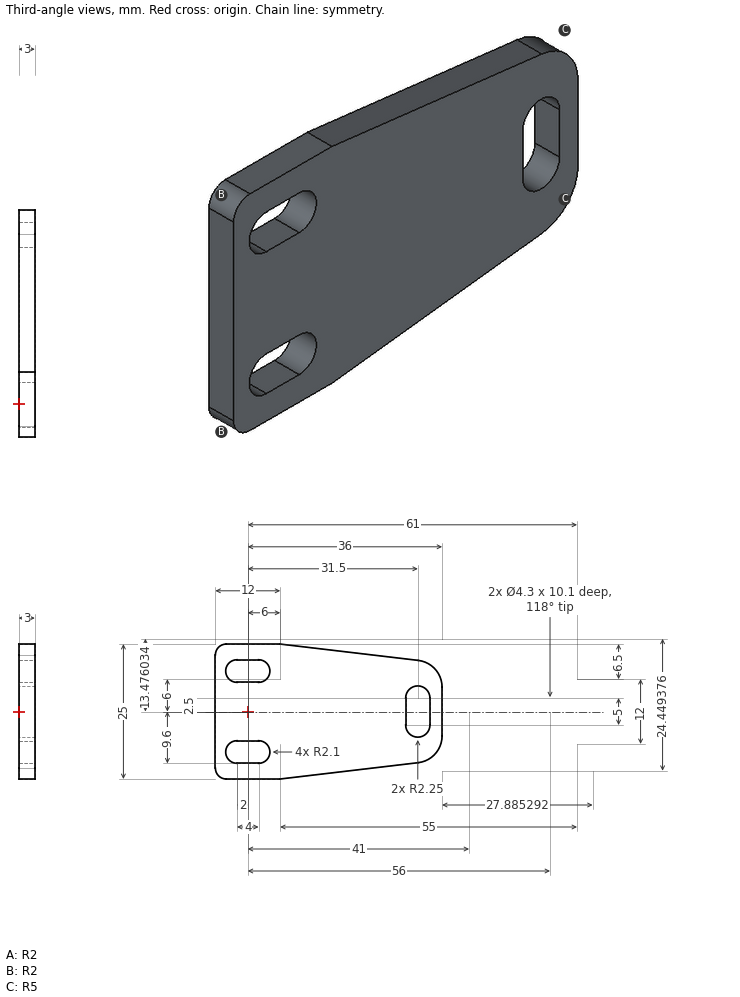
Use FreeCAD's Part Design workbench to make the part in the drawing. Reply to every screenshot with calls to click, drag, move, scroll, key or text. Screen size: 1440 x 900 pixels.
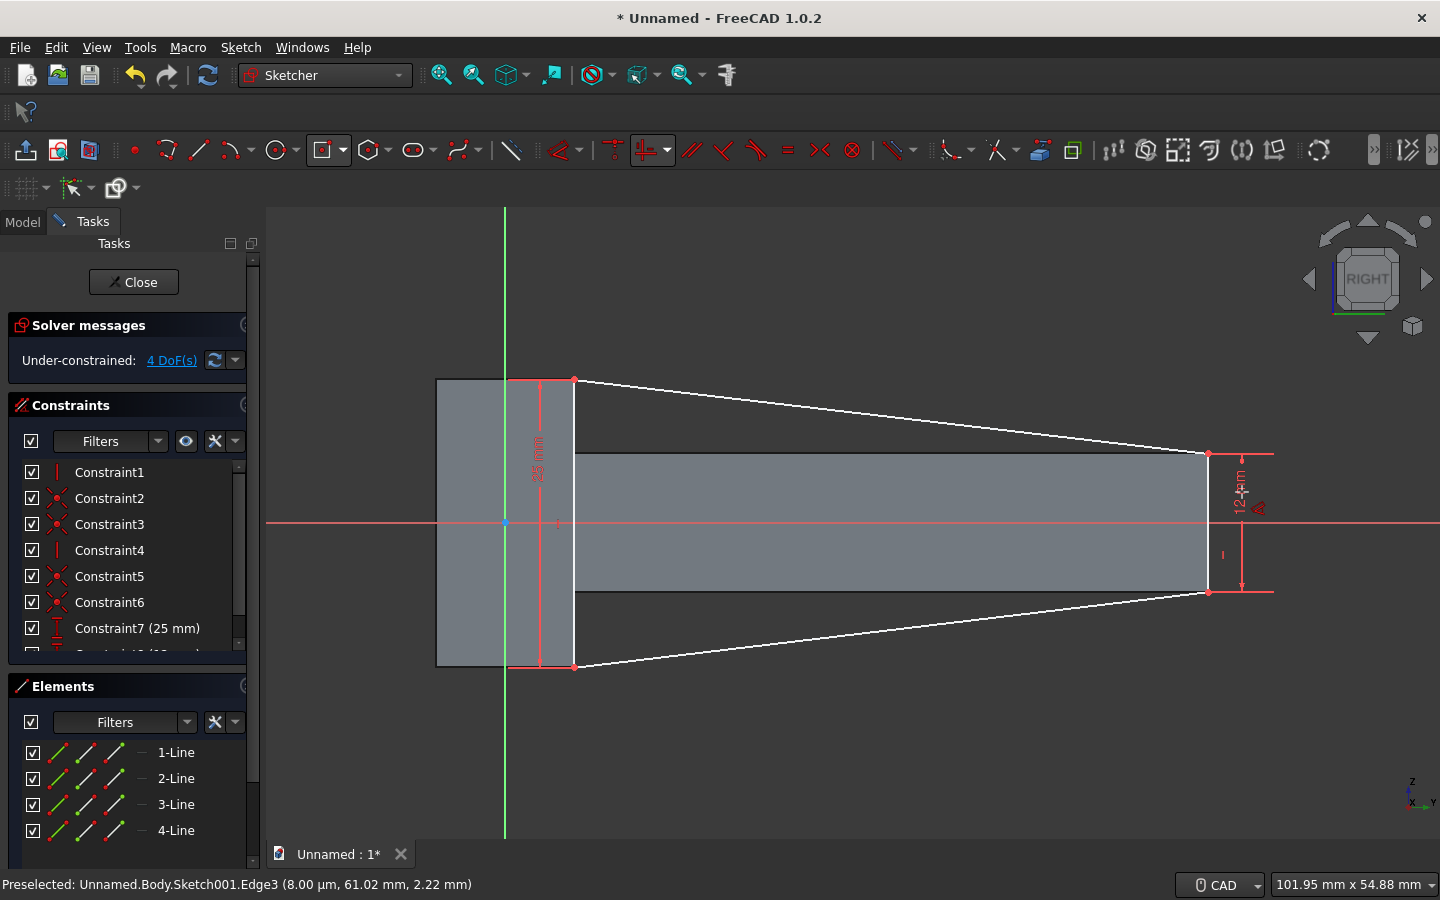
click(574, 668)
click(540, 702)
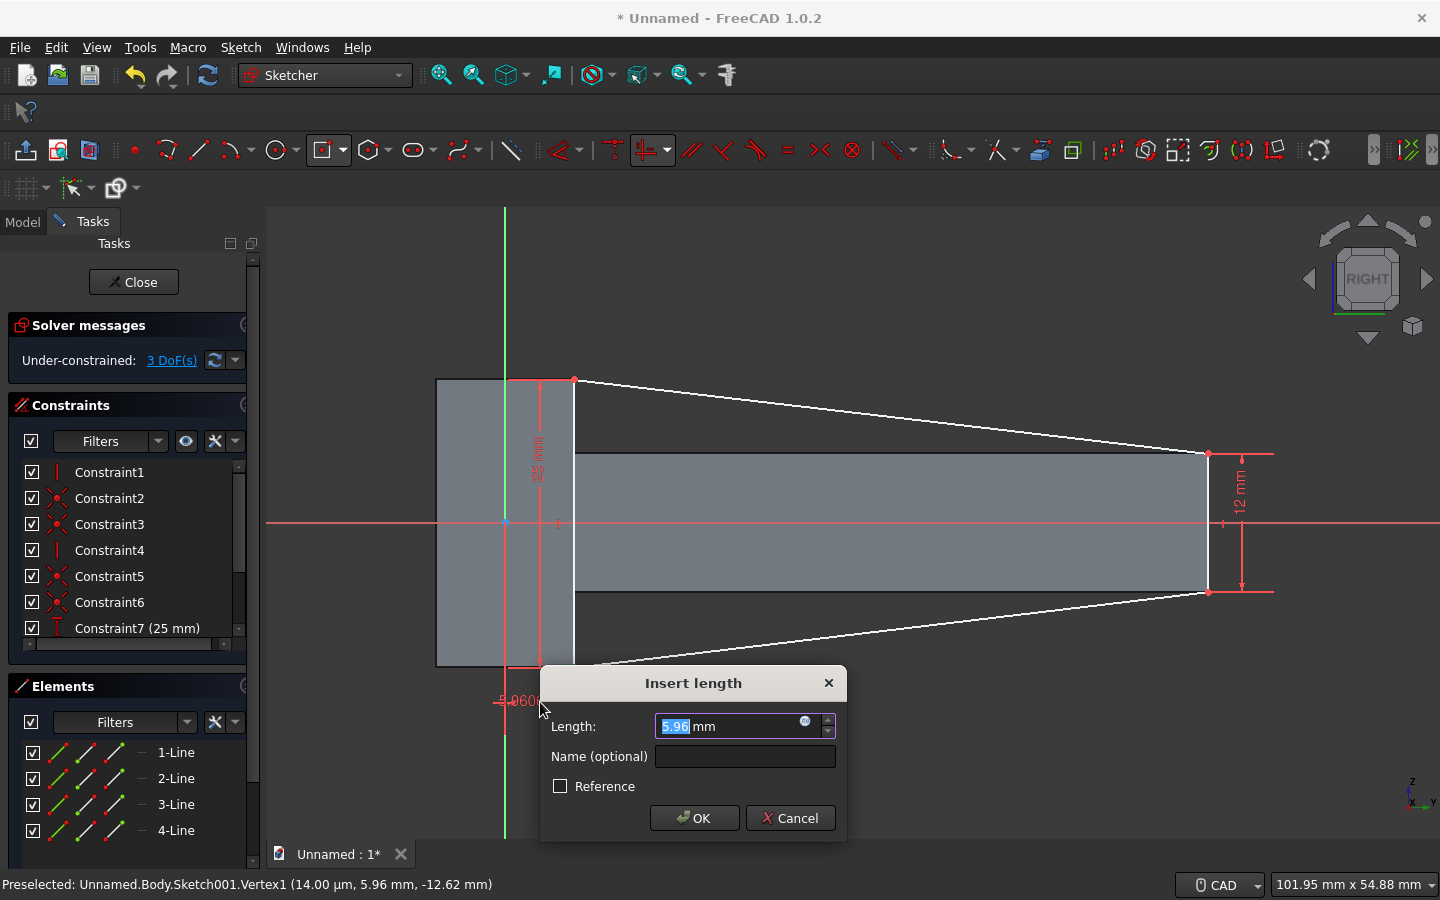
text(6)
key(Return)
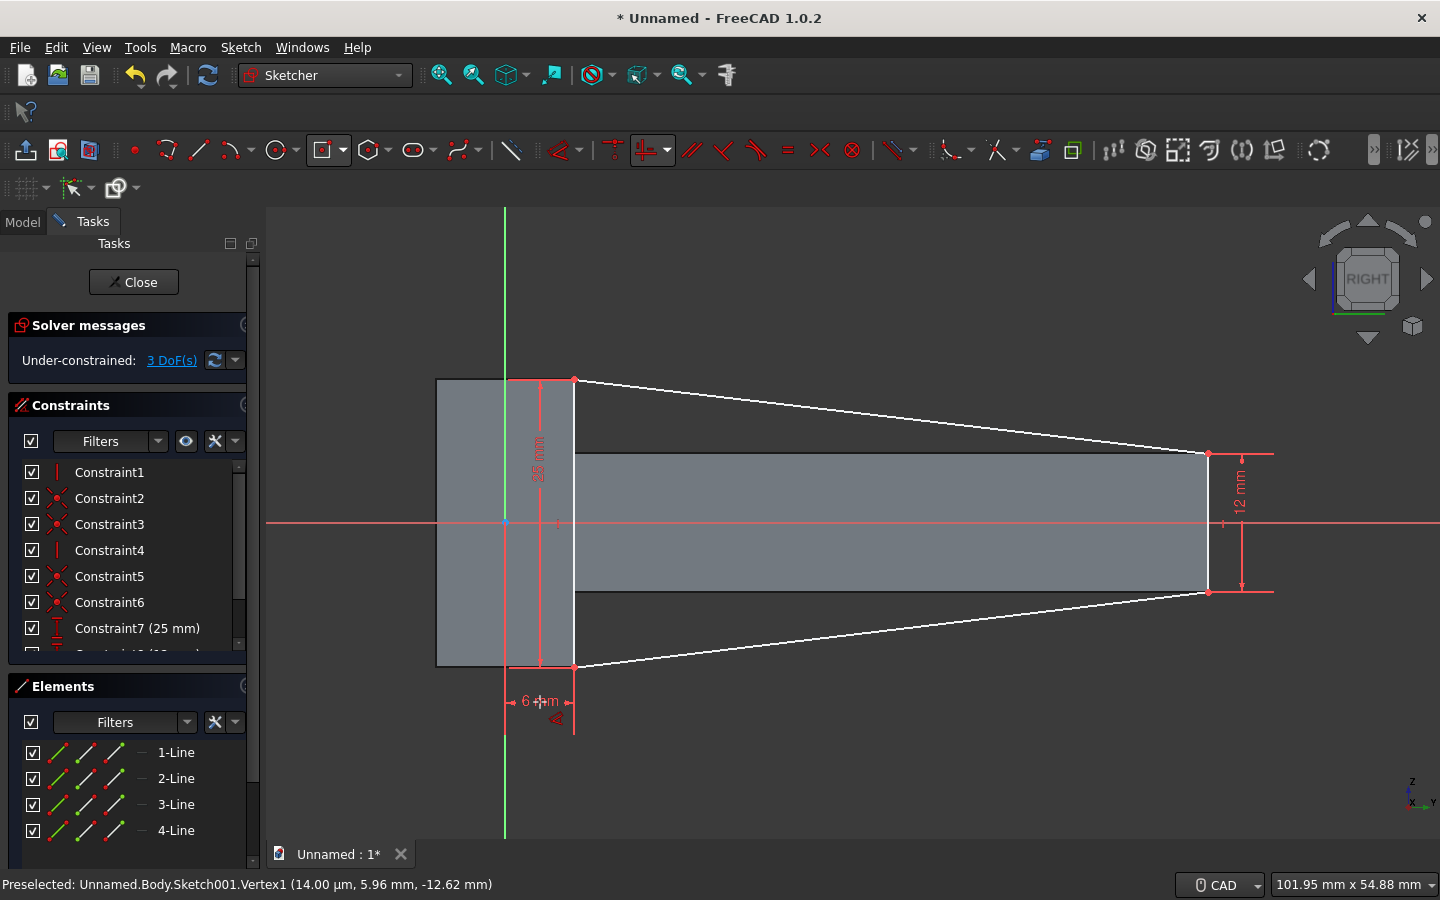
click(1208, 454)
click(1242, 464)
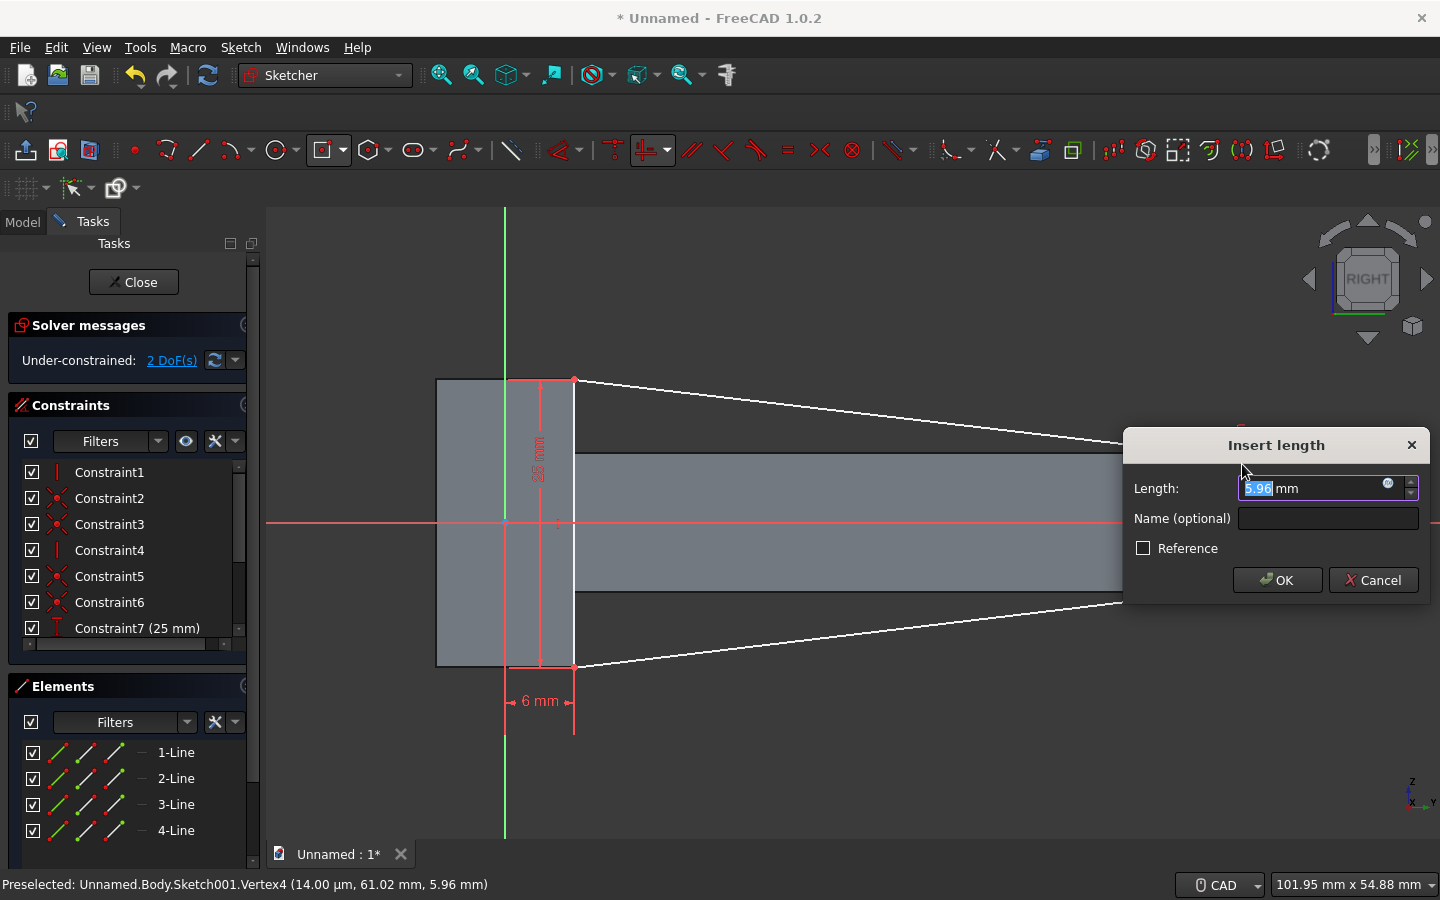
text(6)
key(Return)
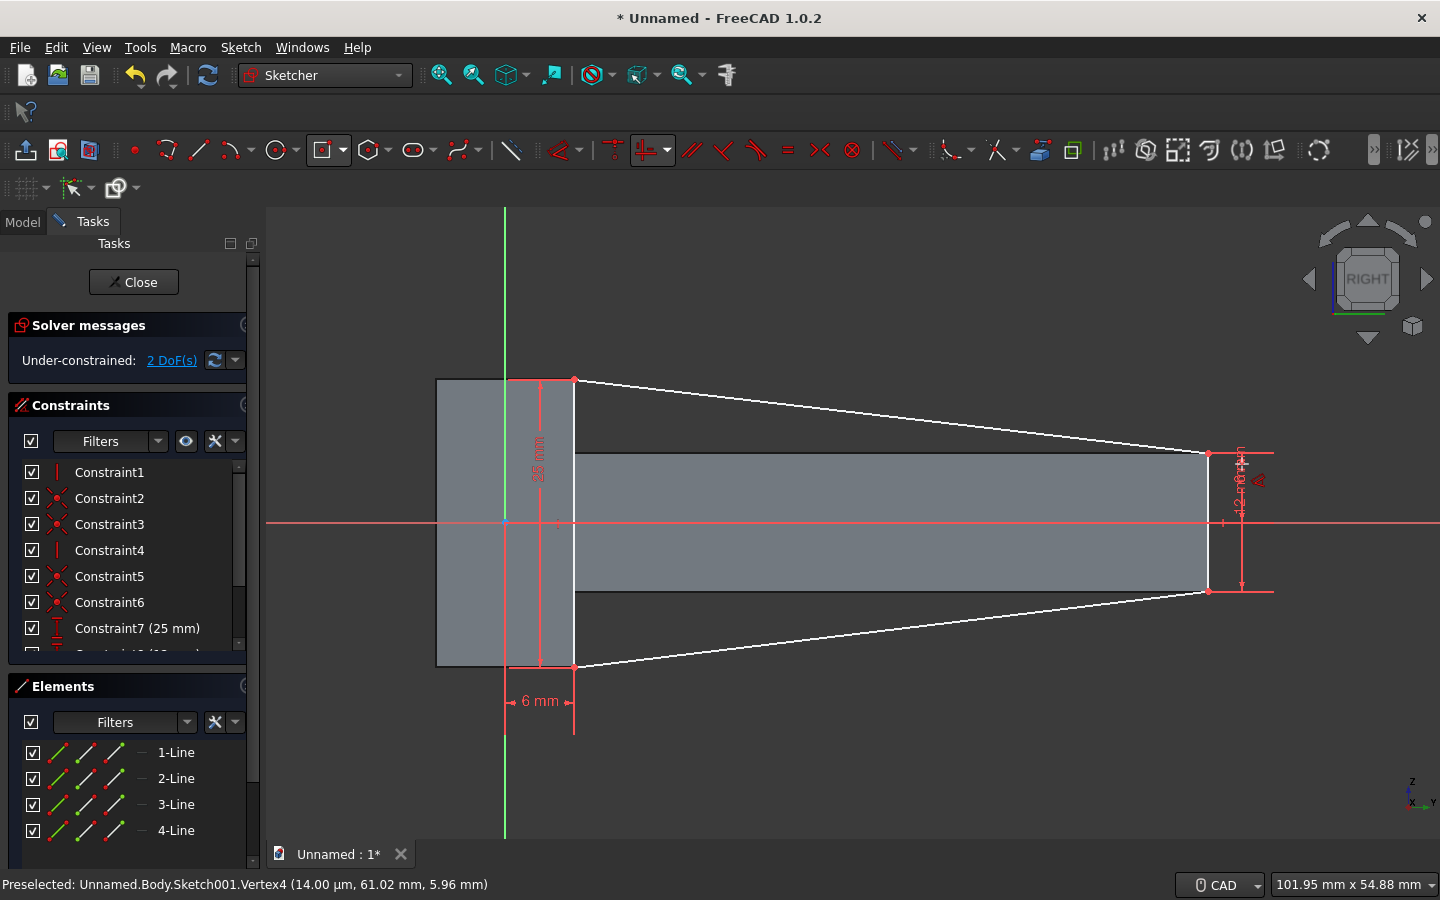
click(1208, 453)
click(695, 419)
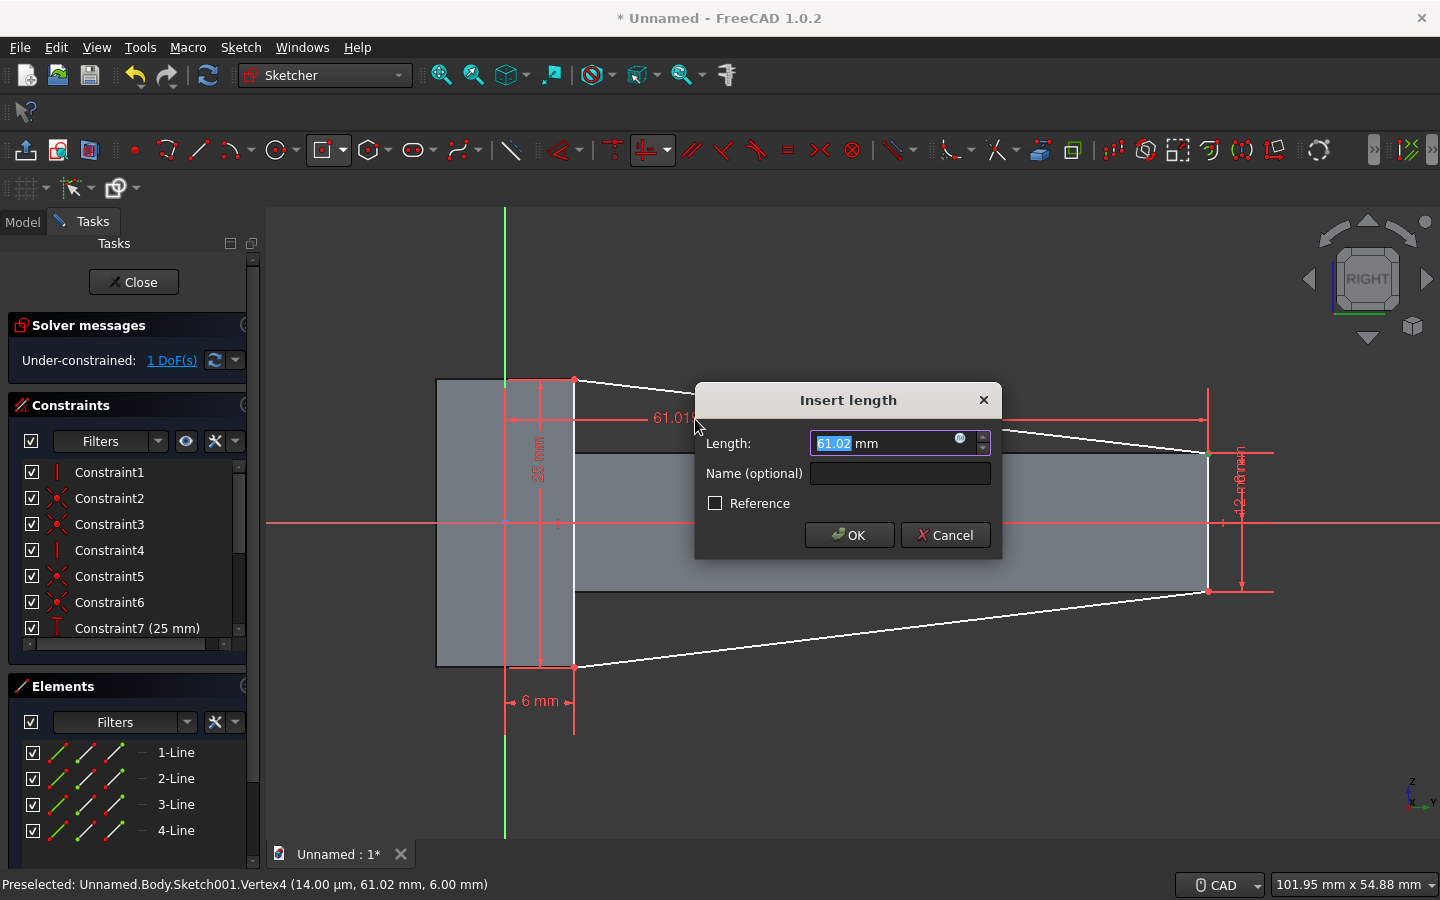
text(61)
key(Return)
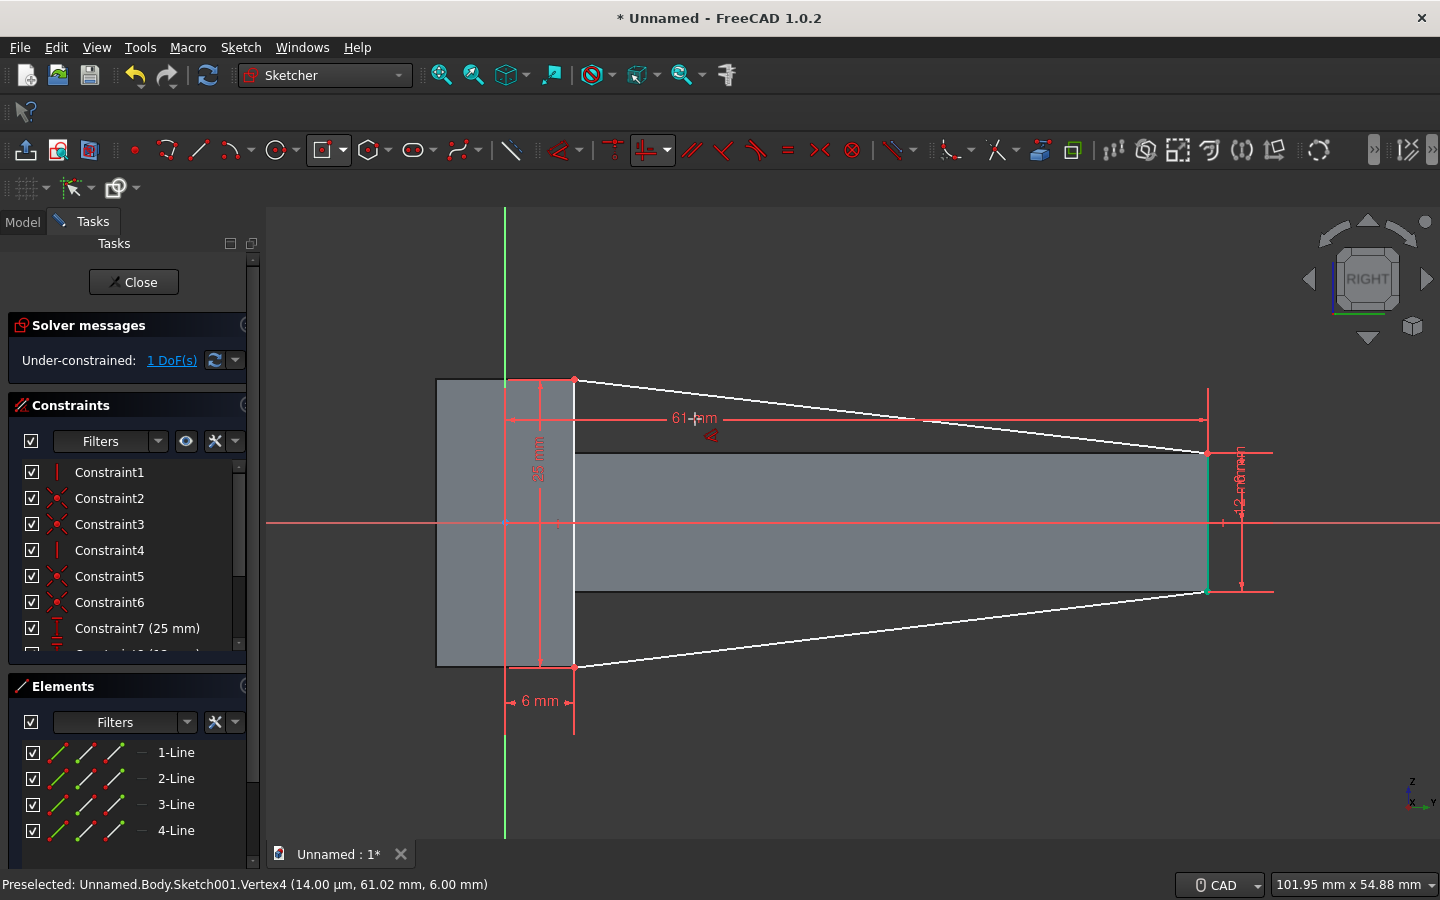
click(764, 402)
click(1242, 417)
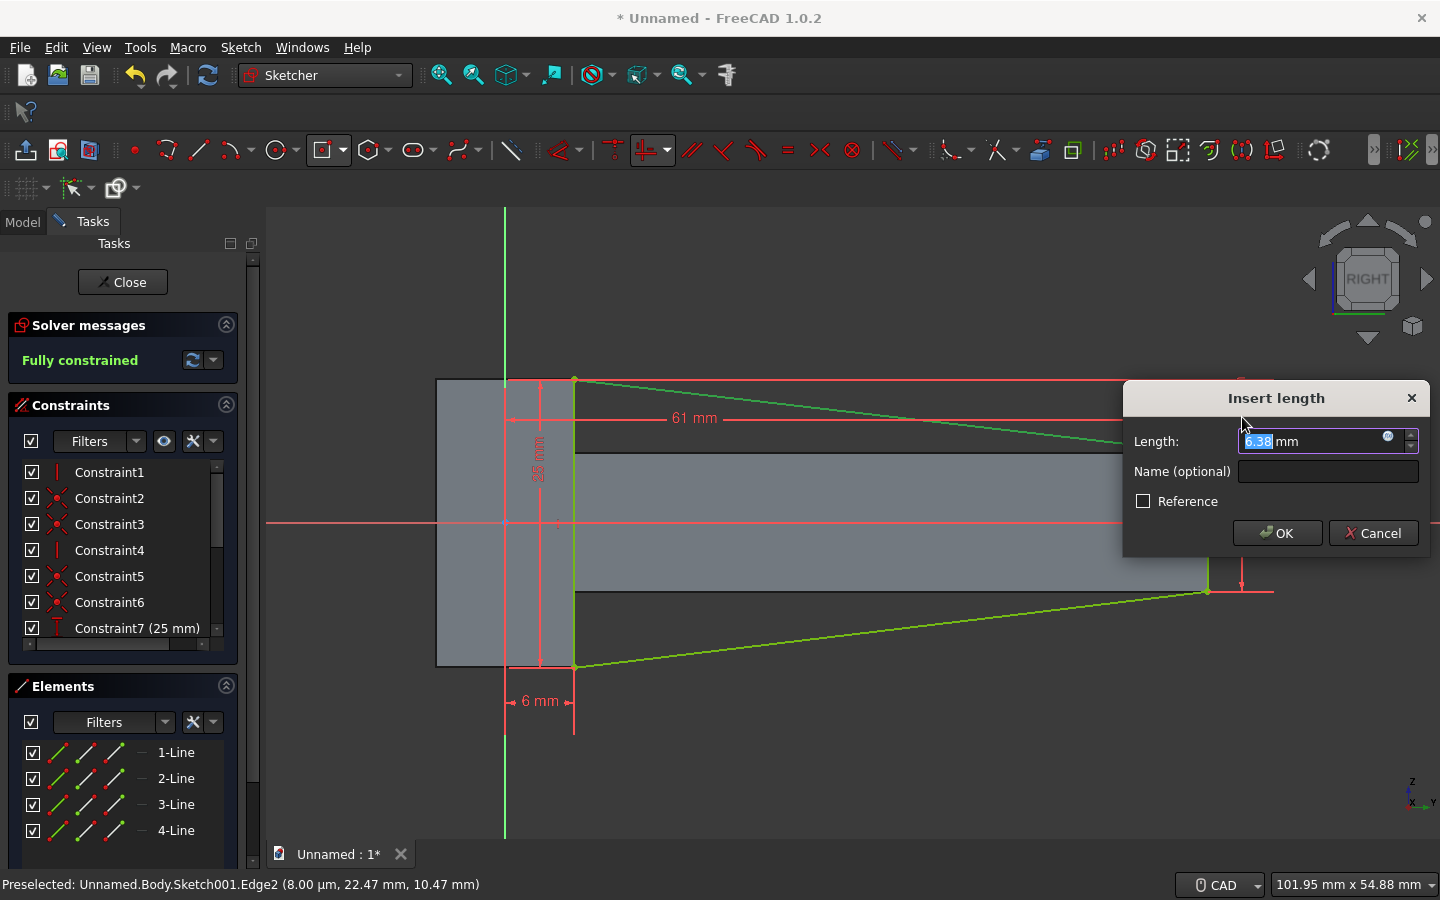
text(6.5)
key(Return)
key(Escape)